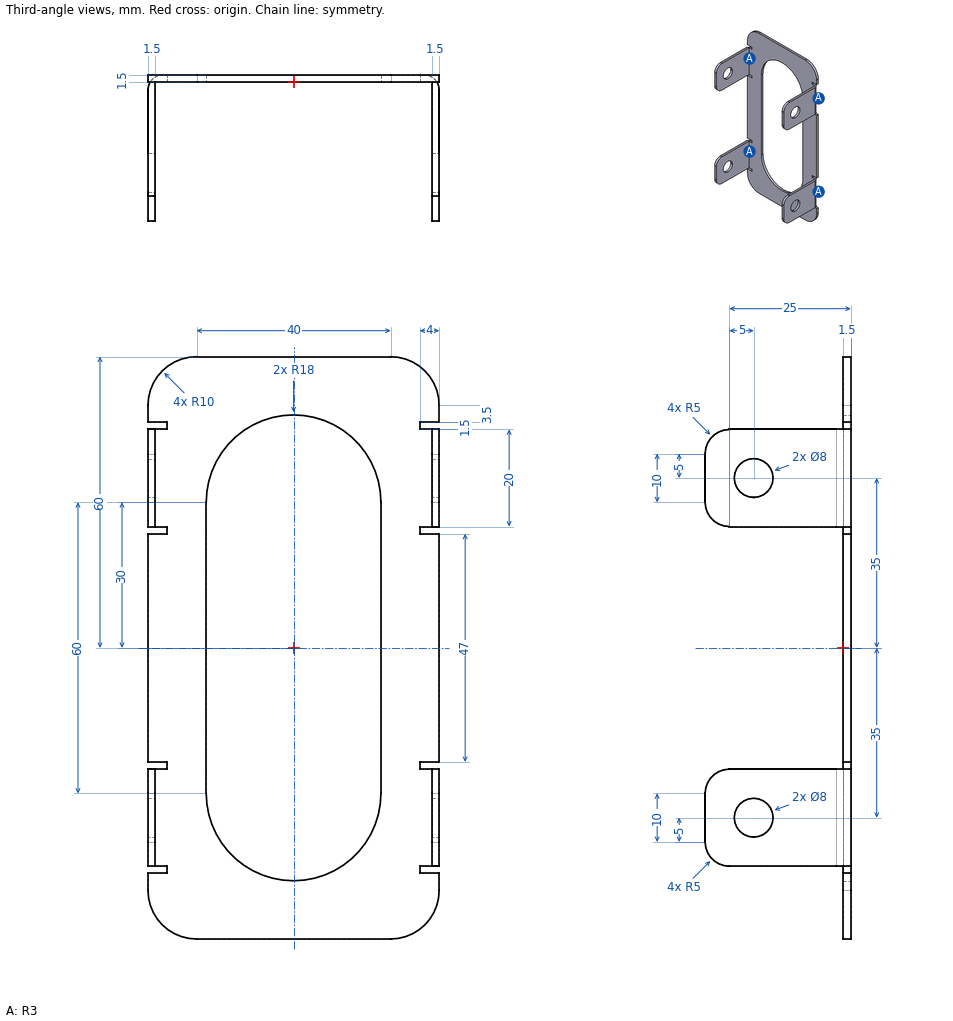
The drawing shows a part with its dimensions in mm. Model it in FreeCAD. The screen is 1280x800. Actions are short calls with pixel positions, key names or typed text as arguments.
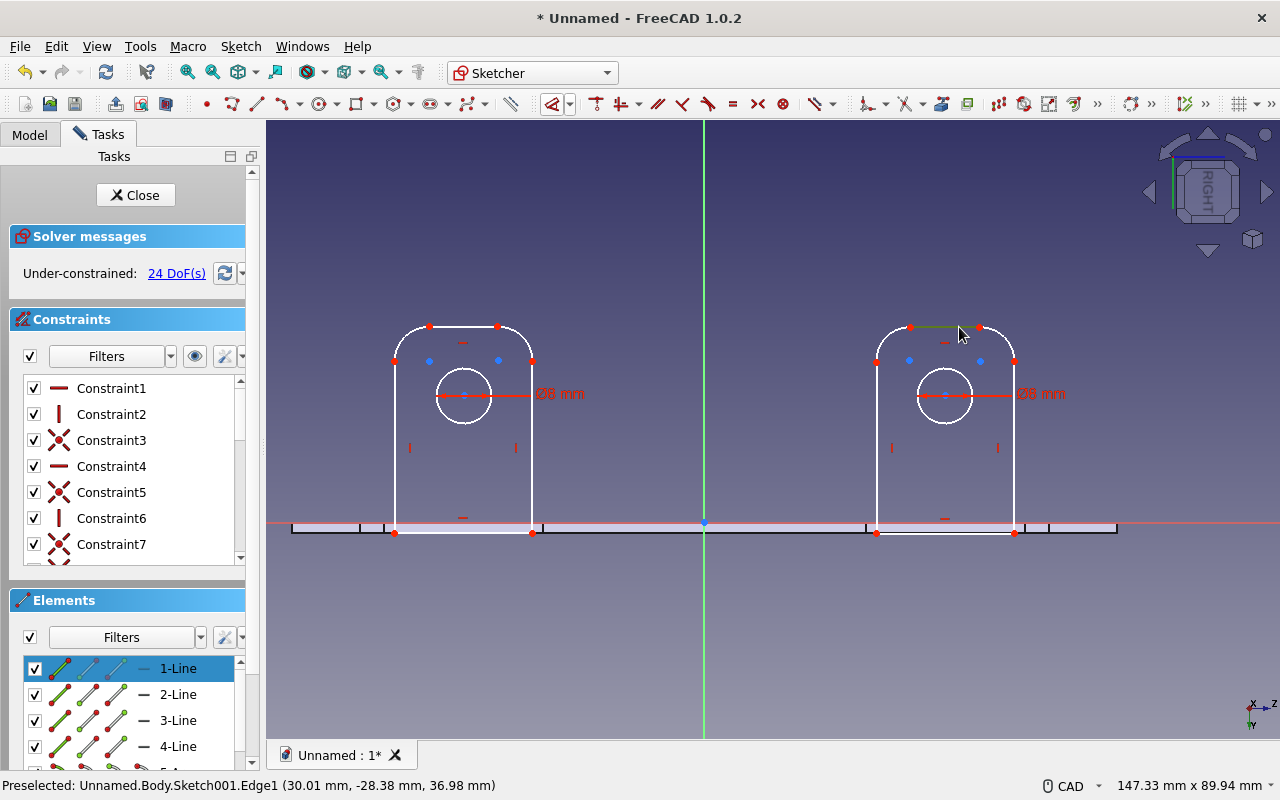
click(895, 331)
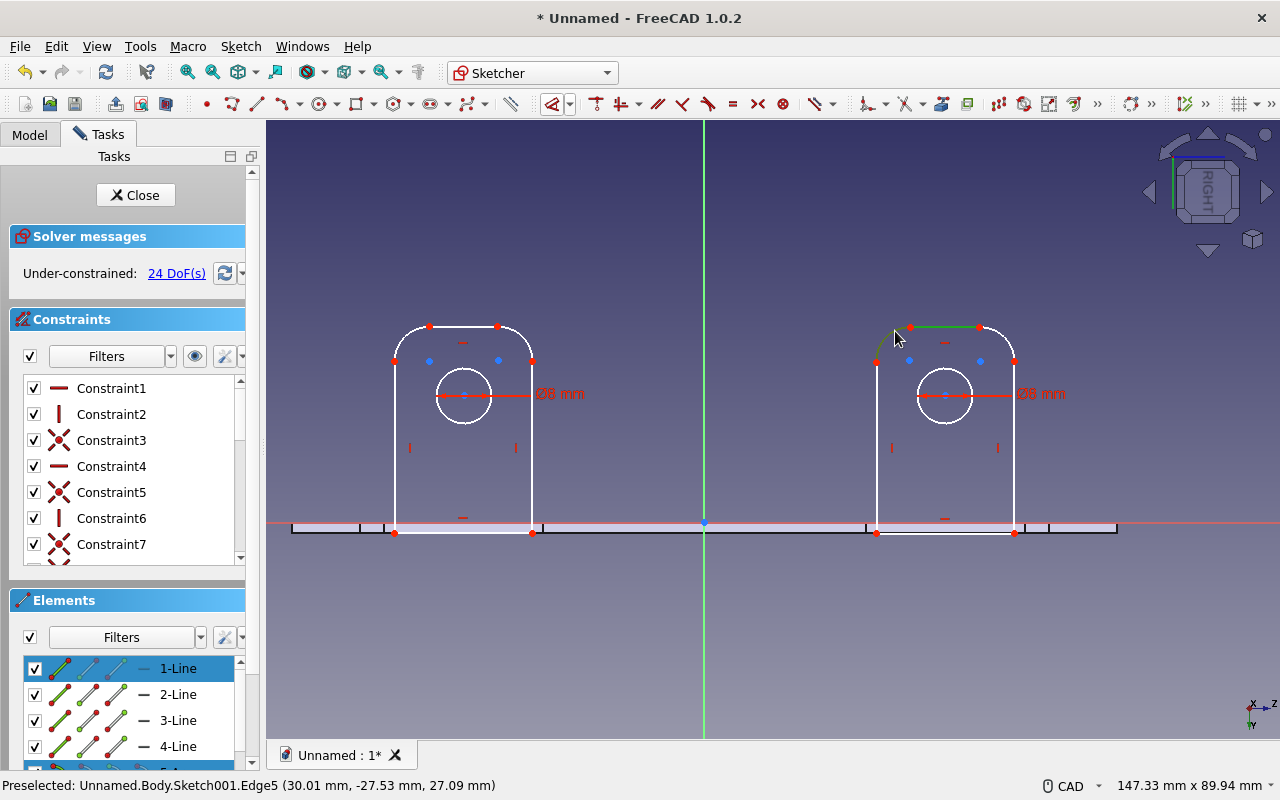
key(t)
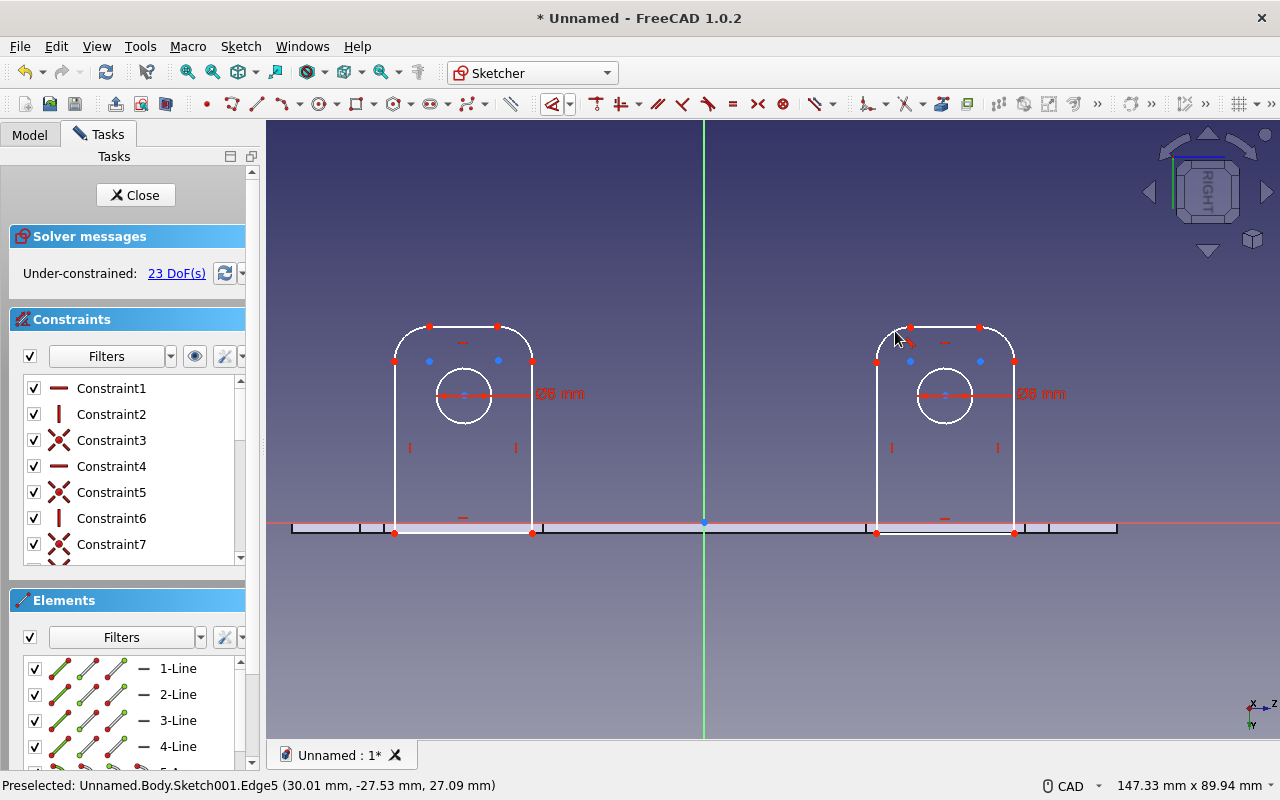
click(959, 327)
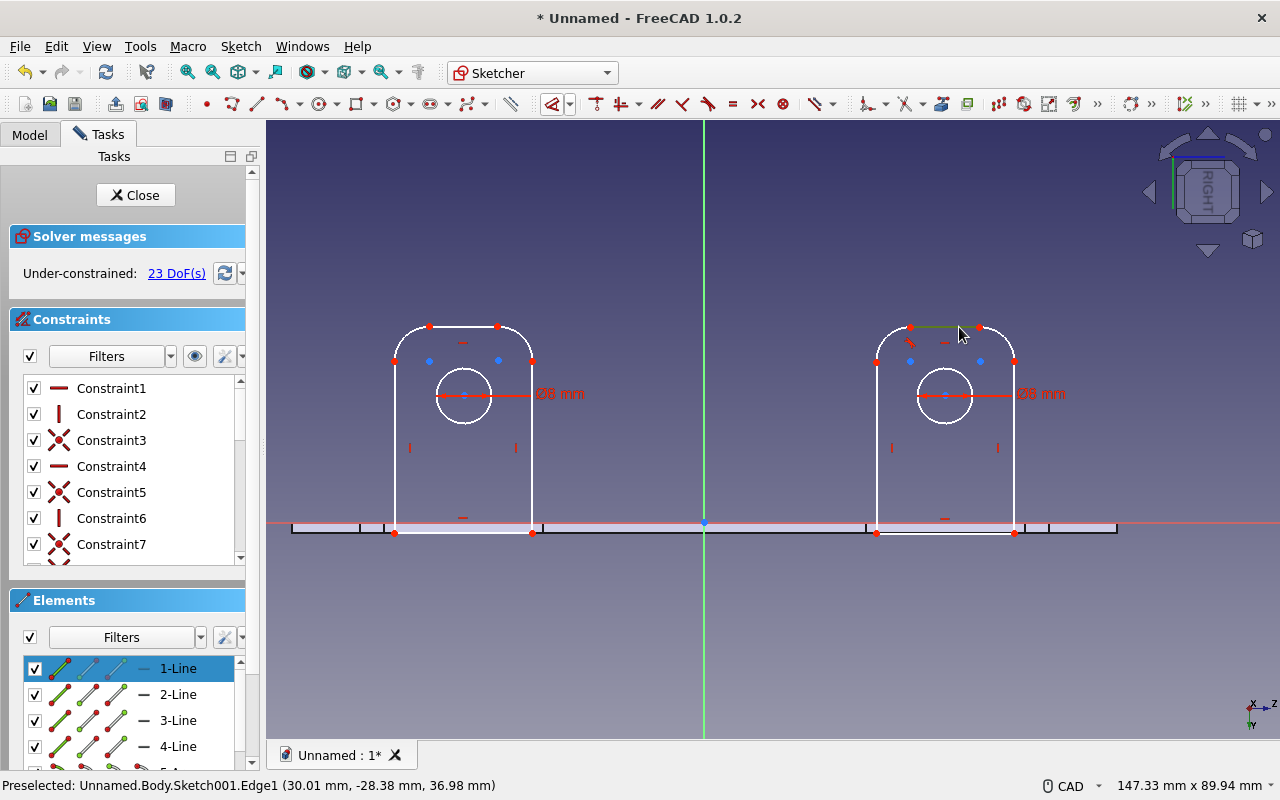
click(1011, 346)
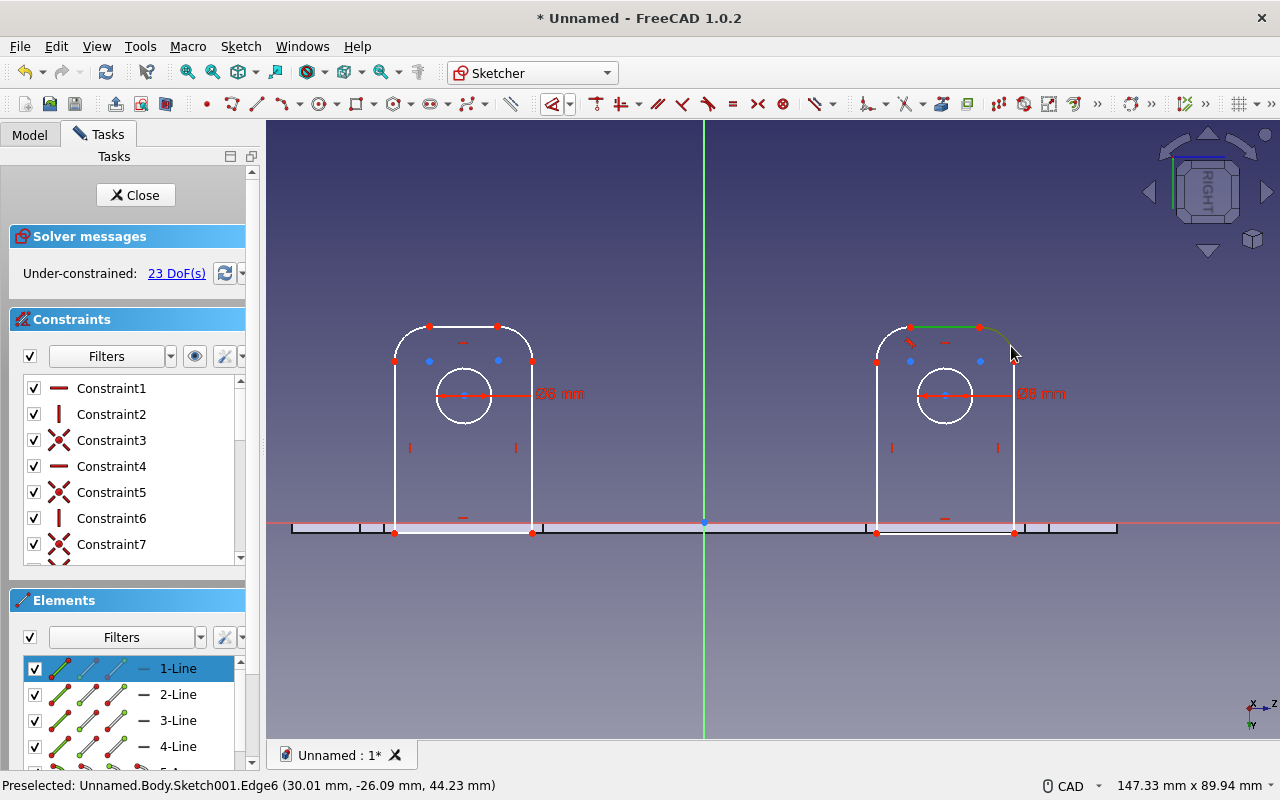
click(708, 104)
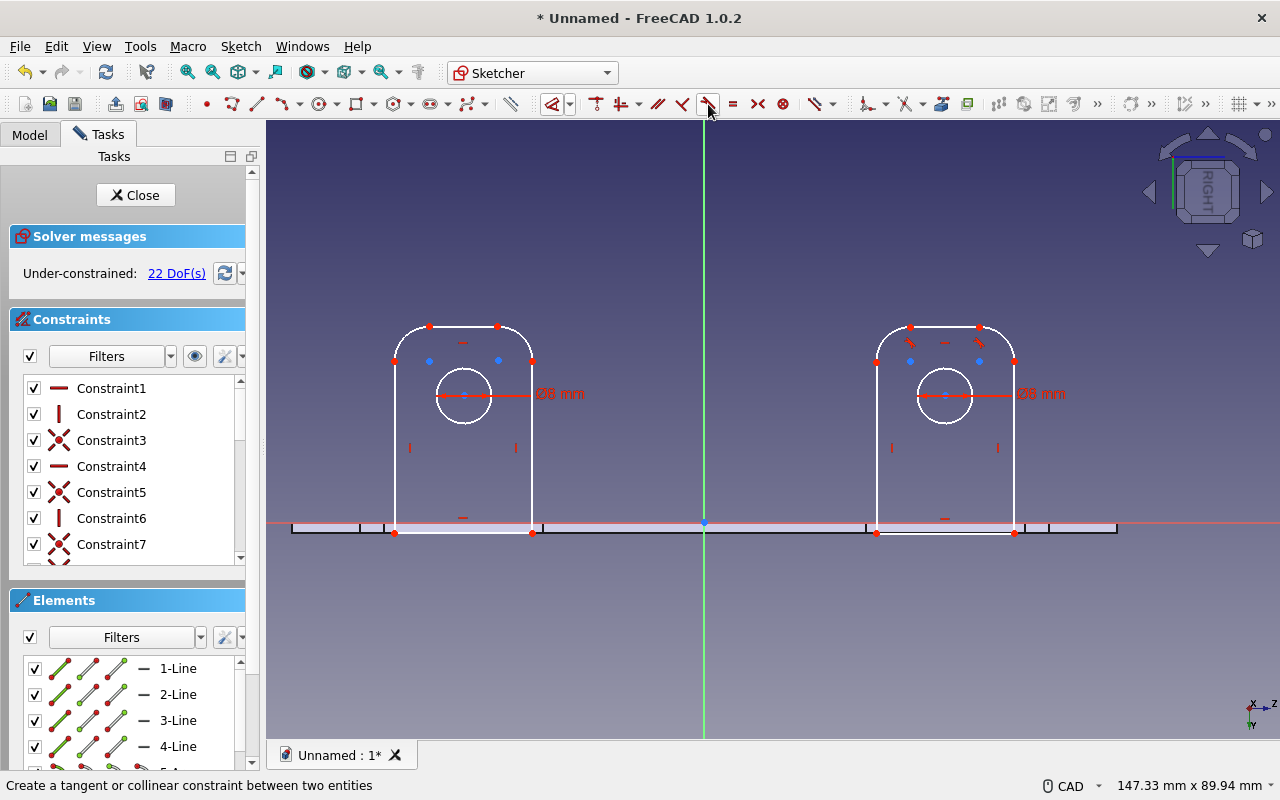
click(877, 414)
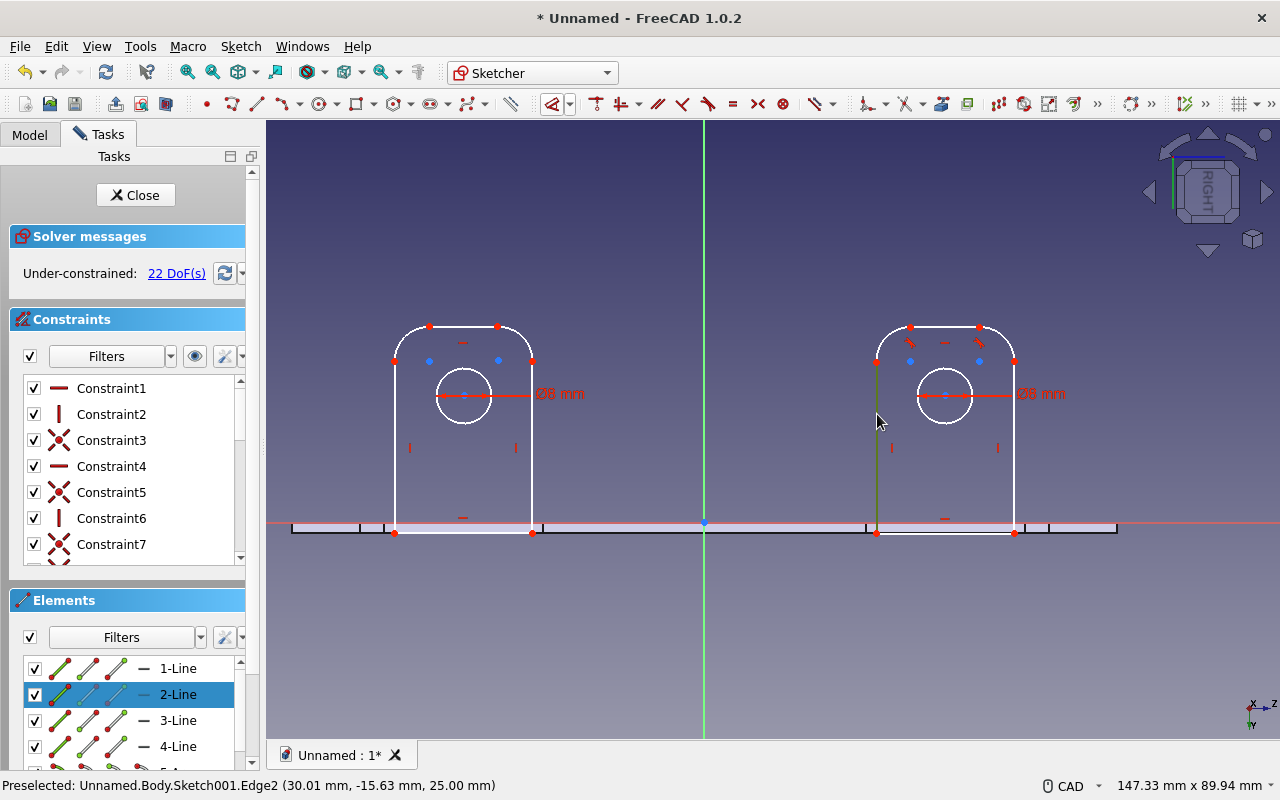
click(895, 331)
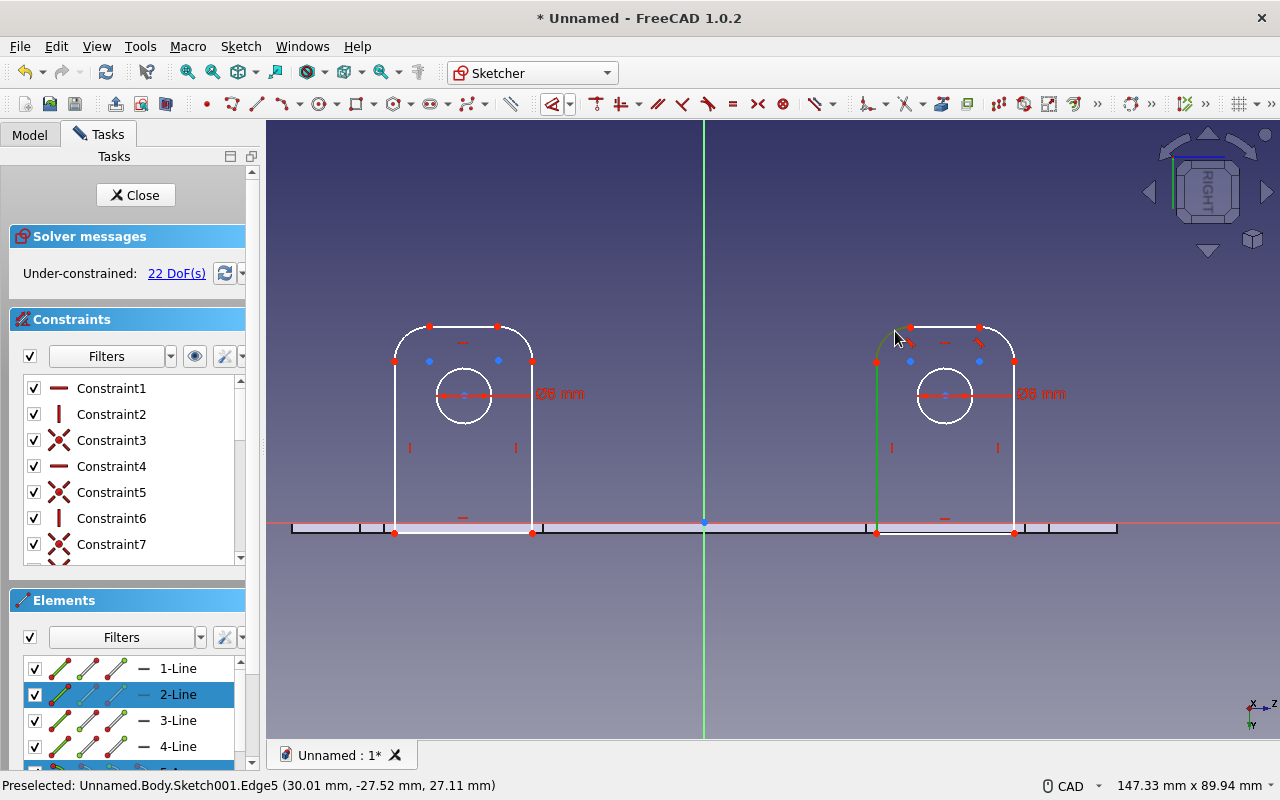
click(708, 104)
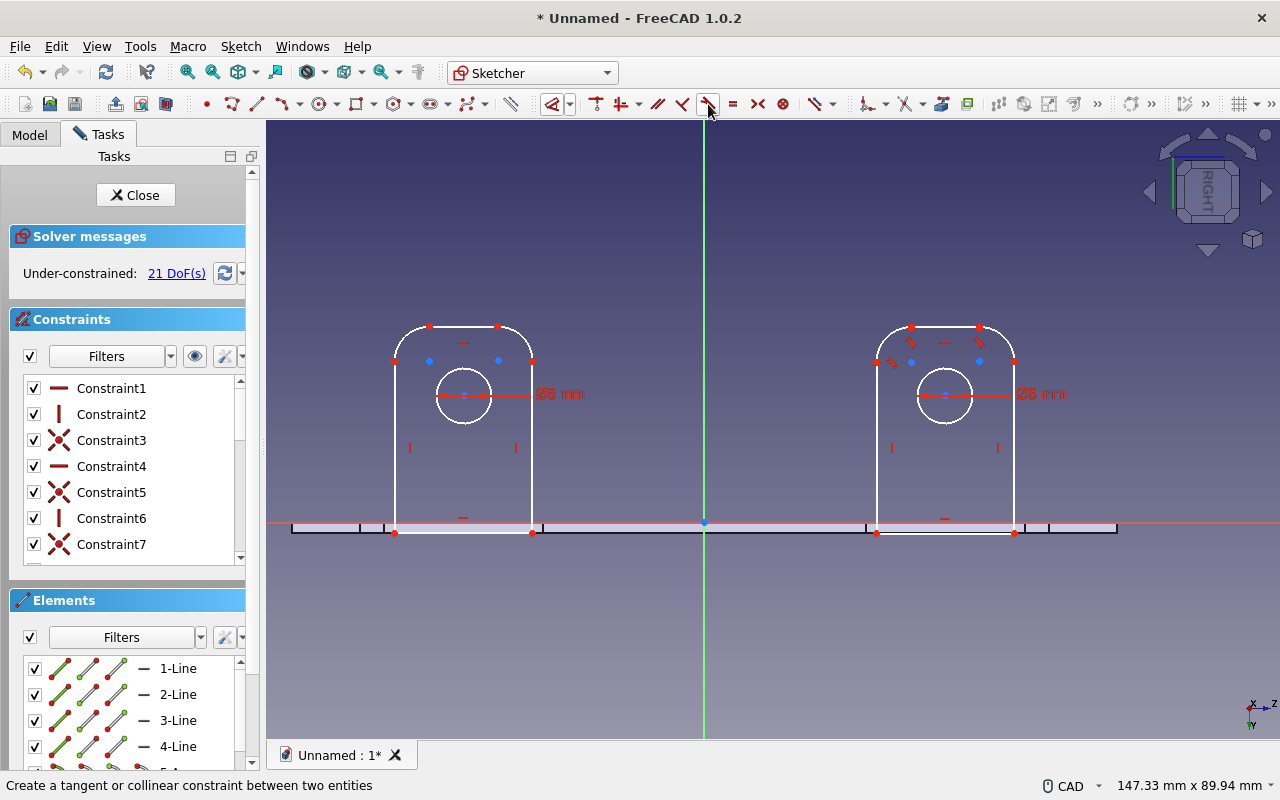
click(1014, 482)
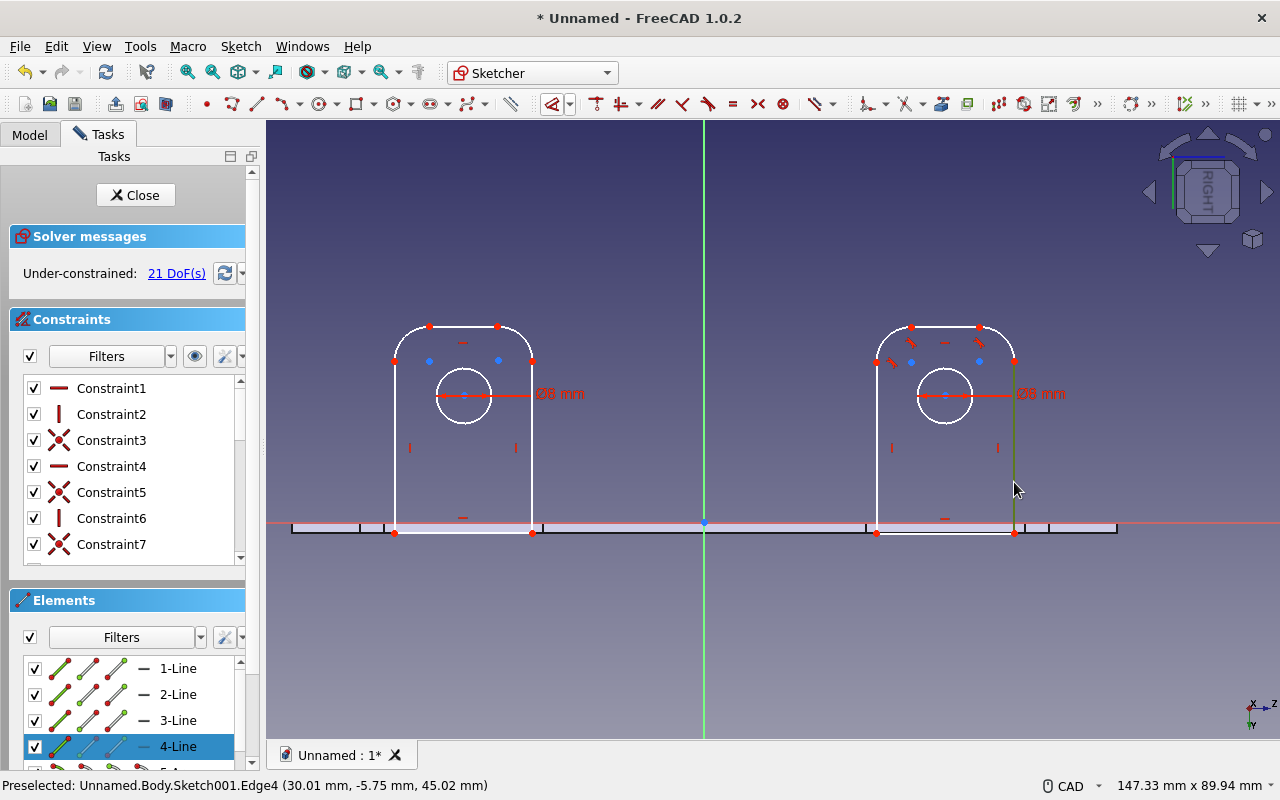
click(1010, 346)